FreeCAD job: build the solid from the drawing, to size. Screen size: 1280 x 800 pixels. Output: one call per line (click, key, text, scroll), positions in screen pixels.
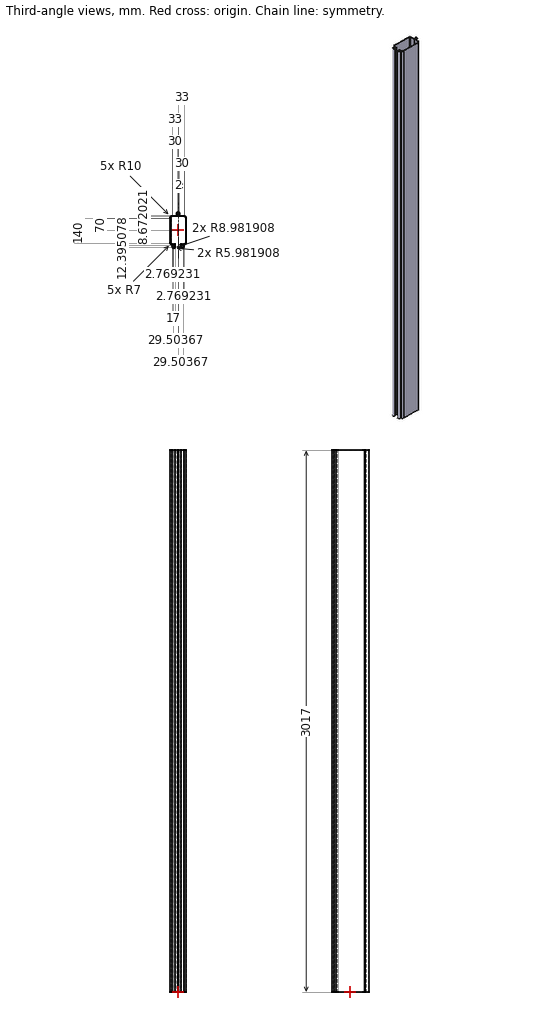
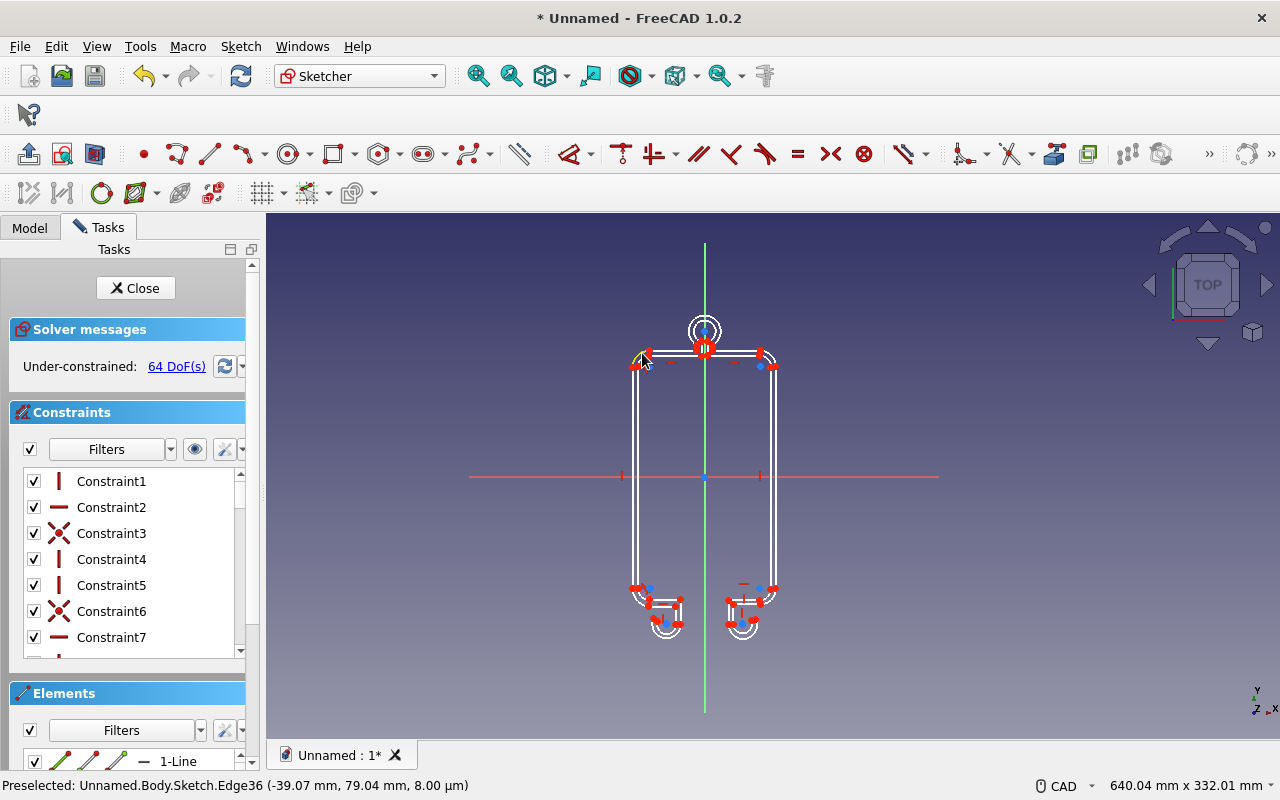
scroll(657, 607, up, 4)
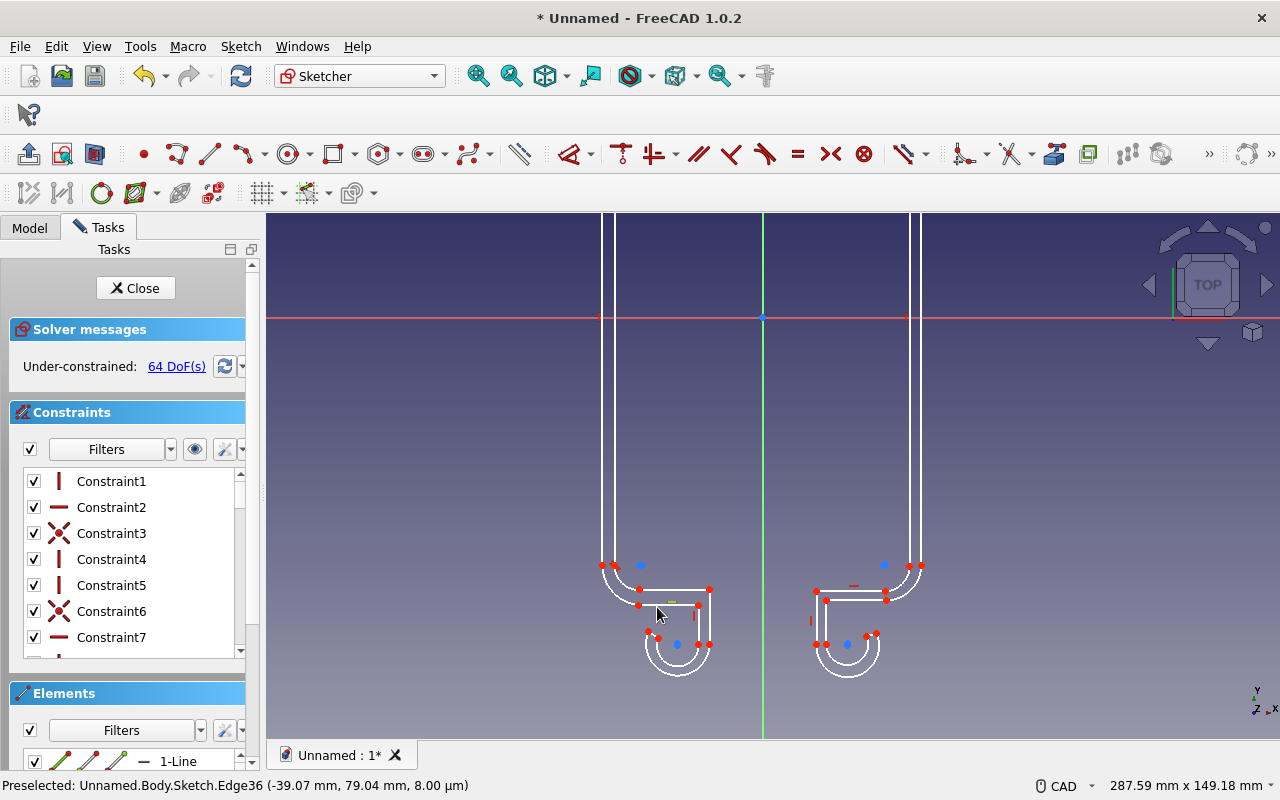
click(656, 605)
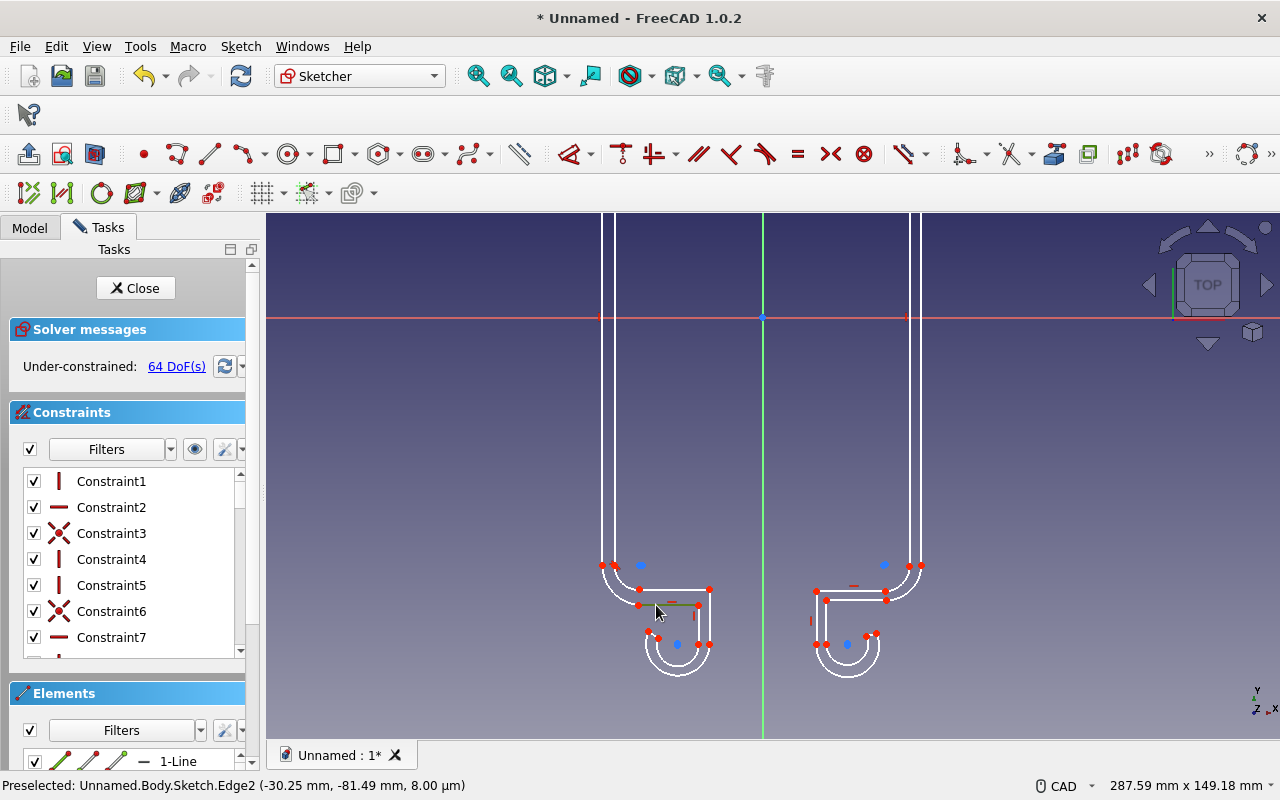
click(606, 582)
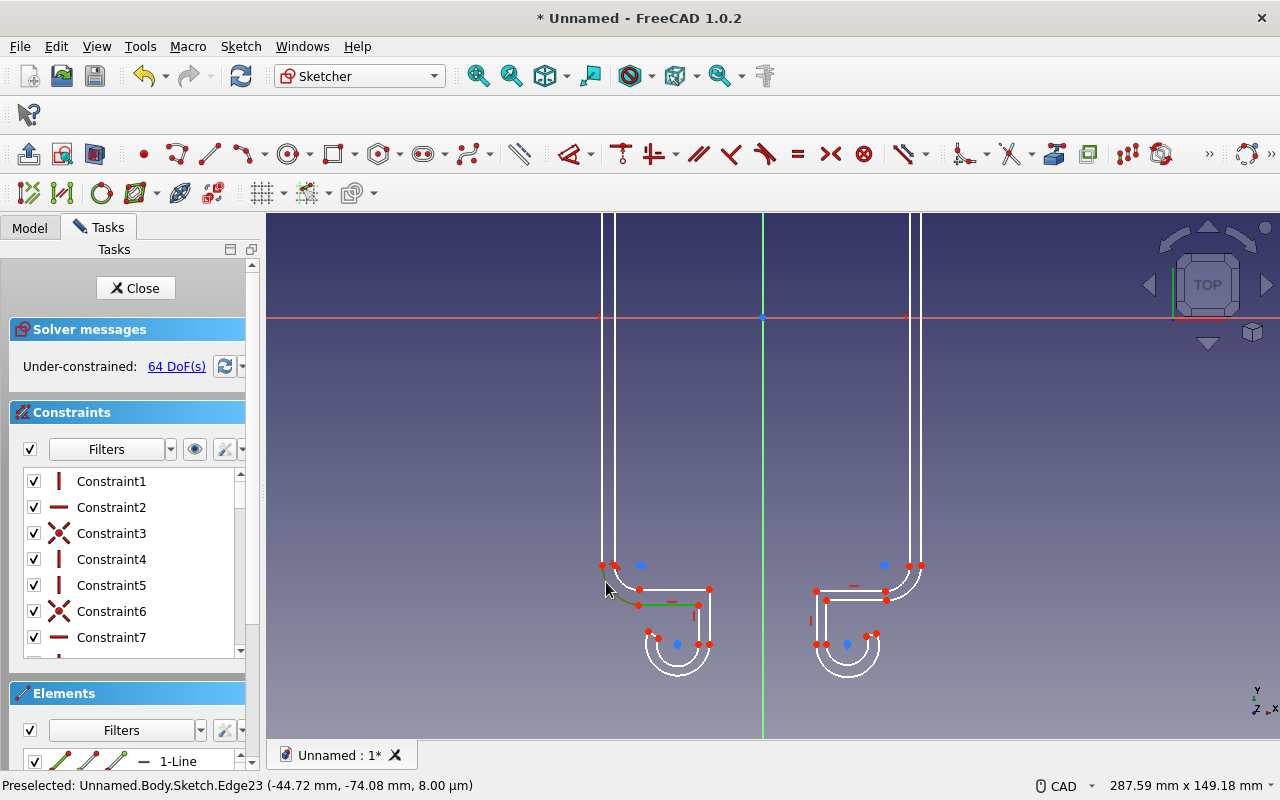
click(765, 154)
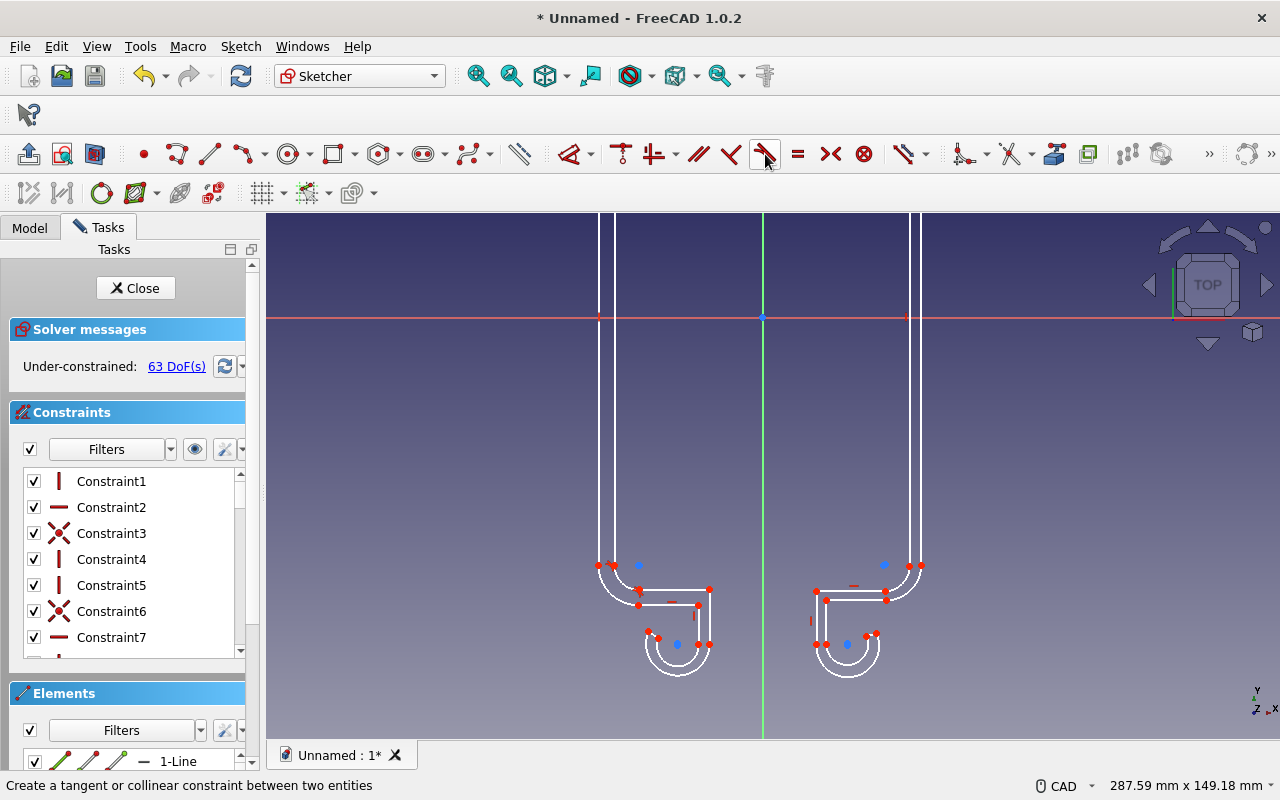
scroll(699, 617, up, 2)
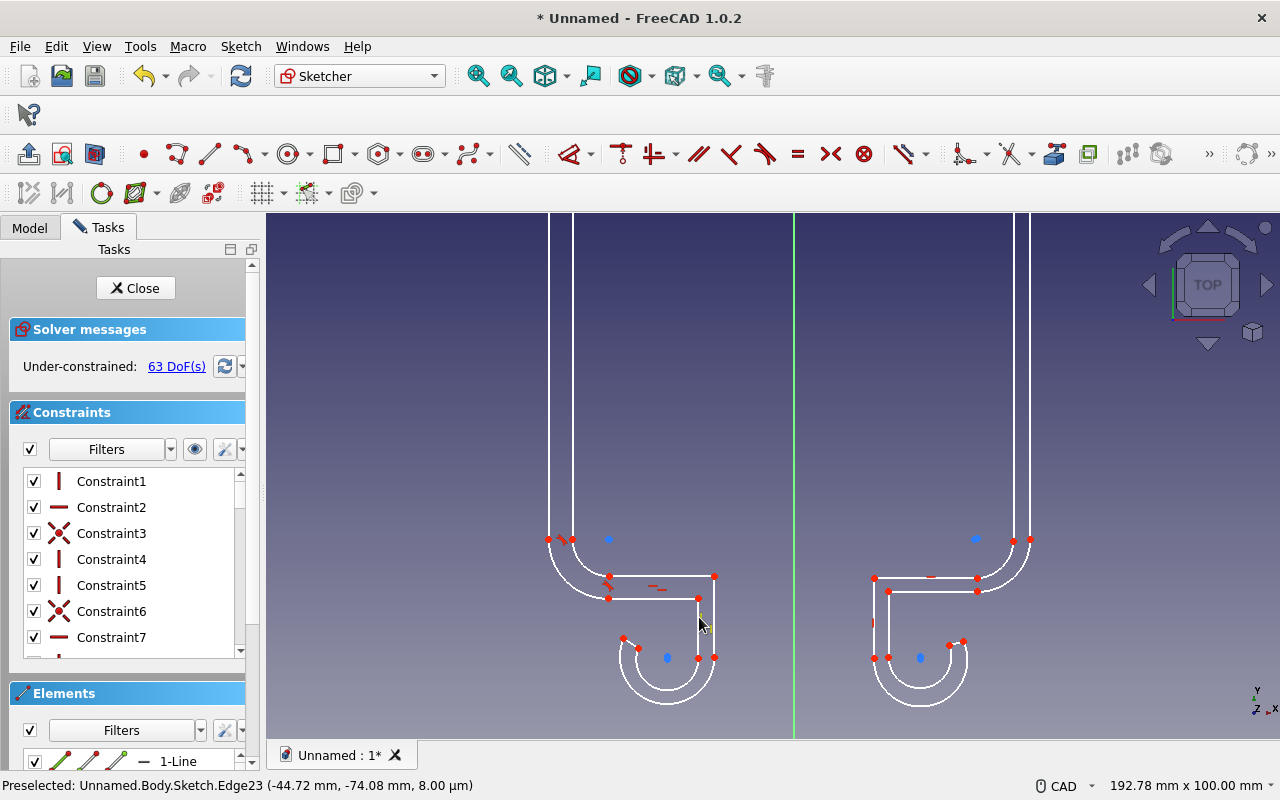
click(698, 640)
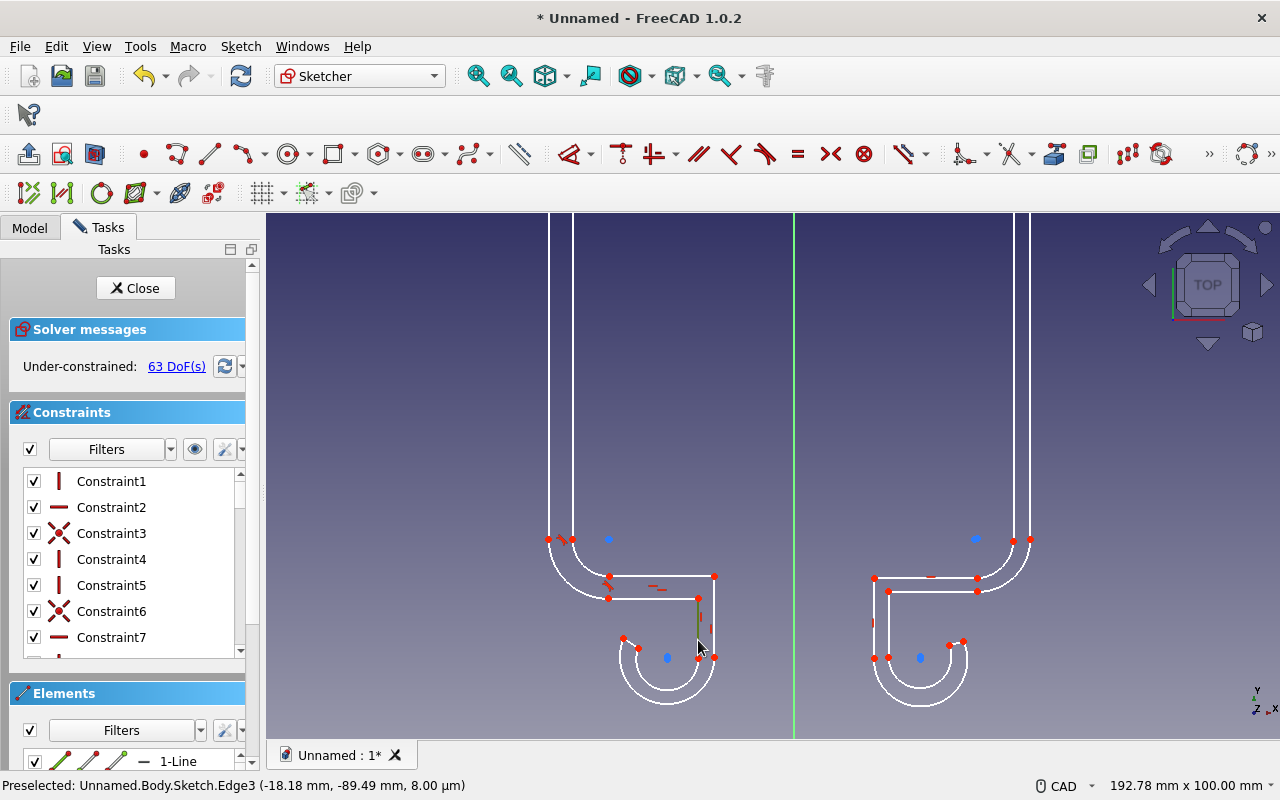
click(643, 679)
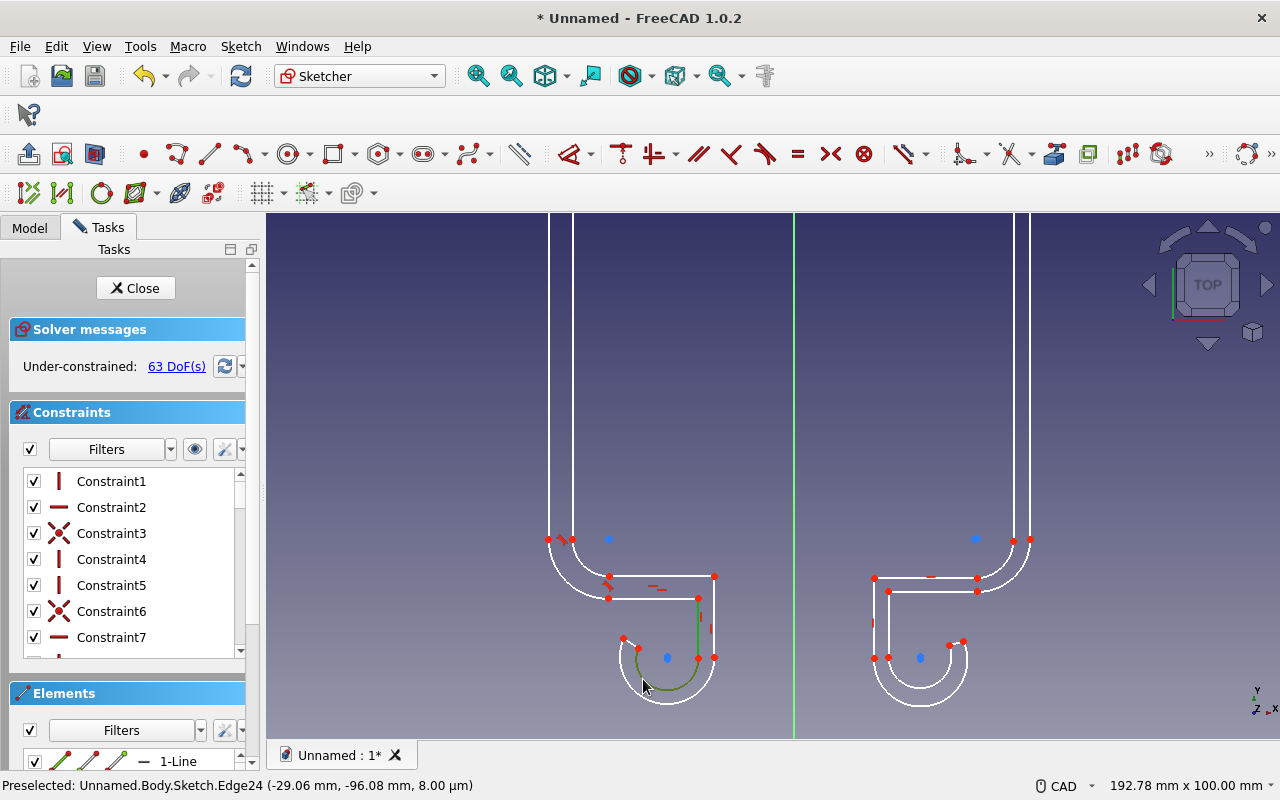
click(765, 154)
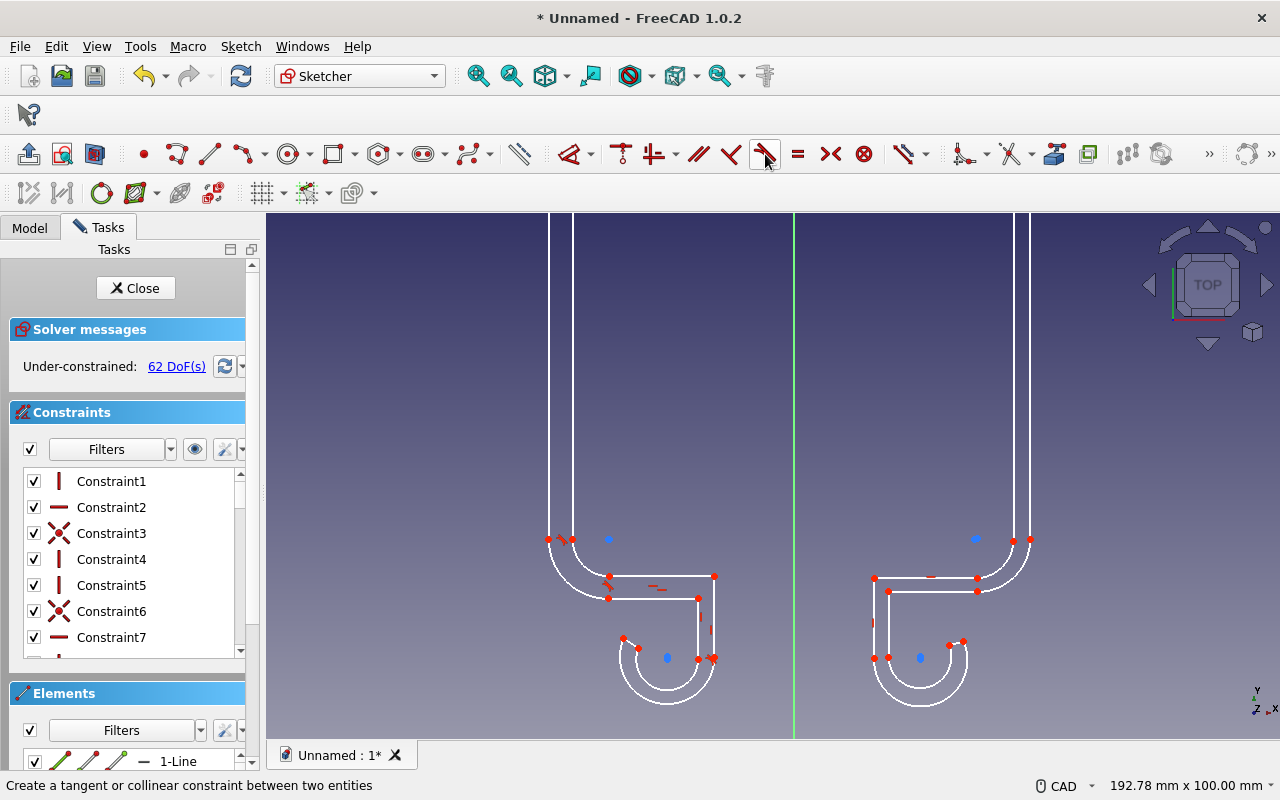
click(714, 601)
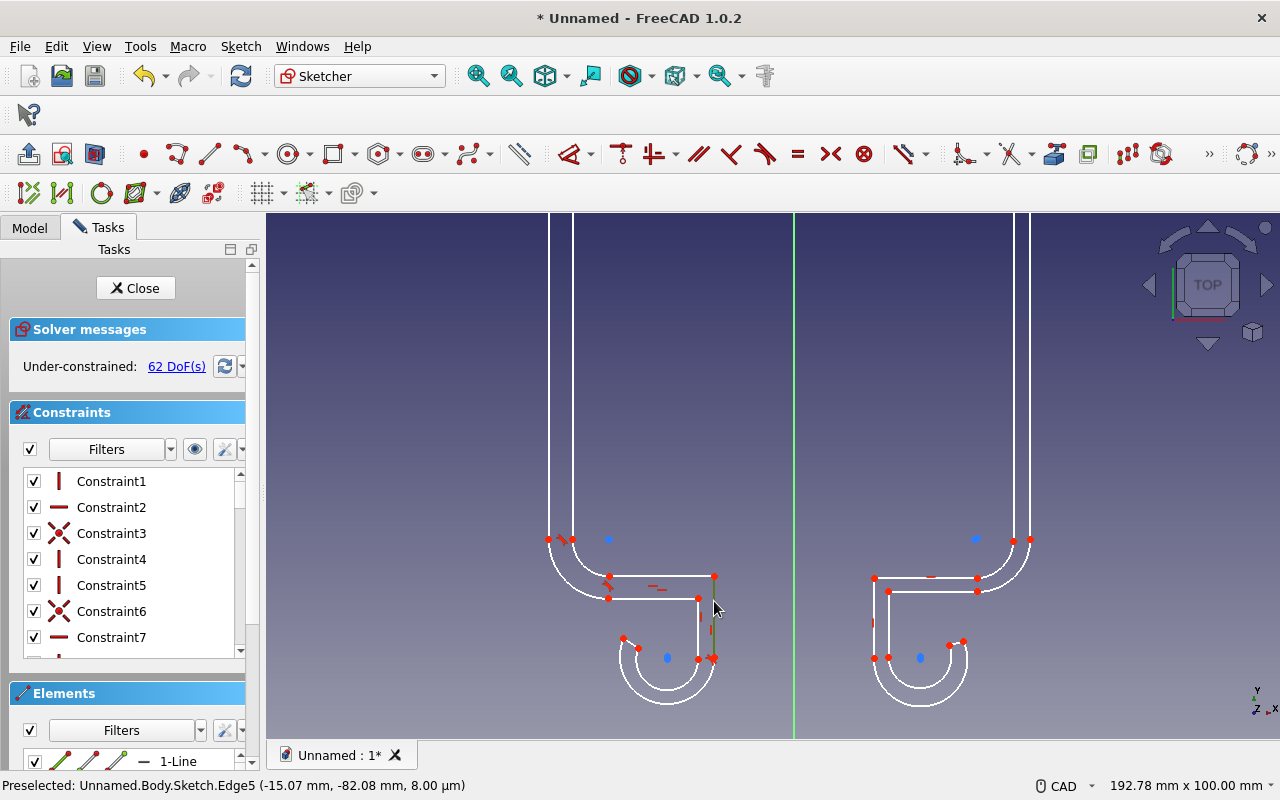
click(630, 686)